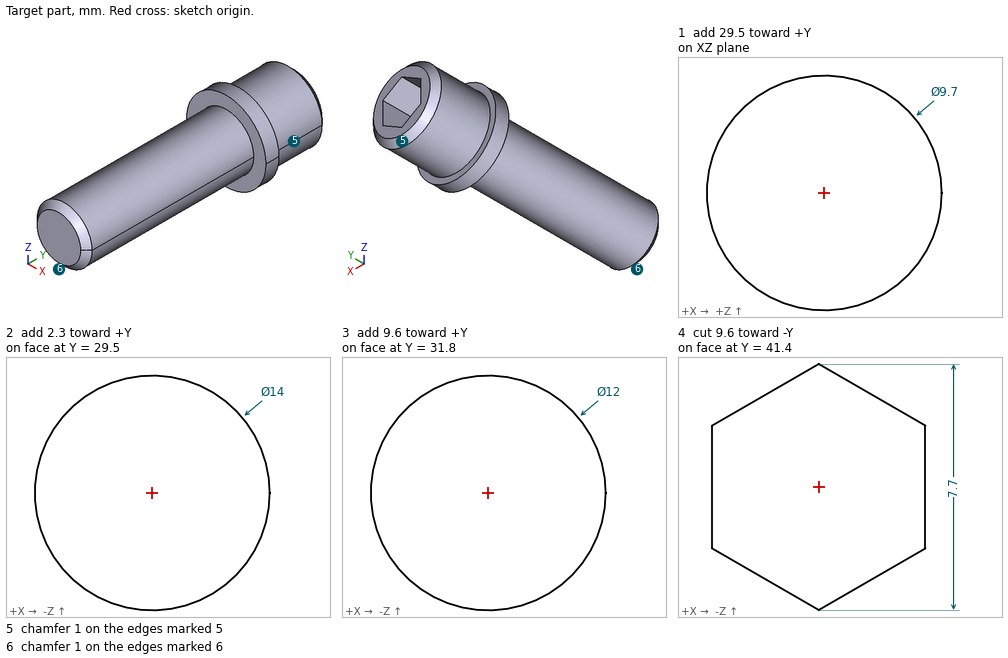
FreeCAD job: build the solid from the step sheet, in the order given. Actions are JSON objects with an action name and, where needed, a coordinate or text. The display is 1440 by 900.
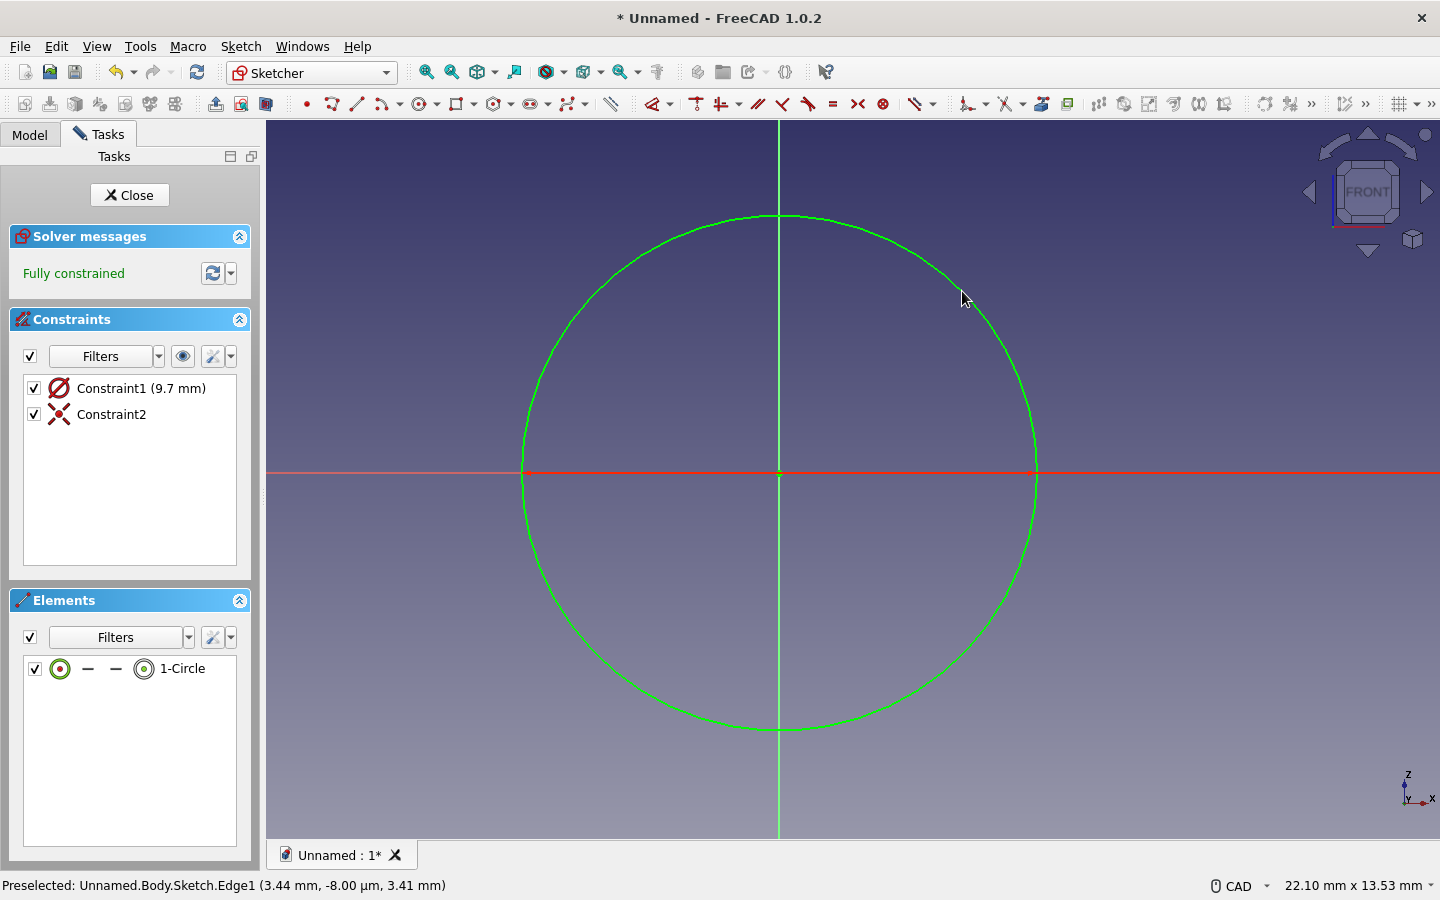
{"action": "left_click", "coordinate": [130, 195]}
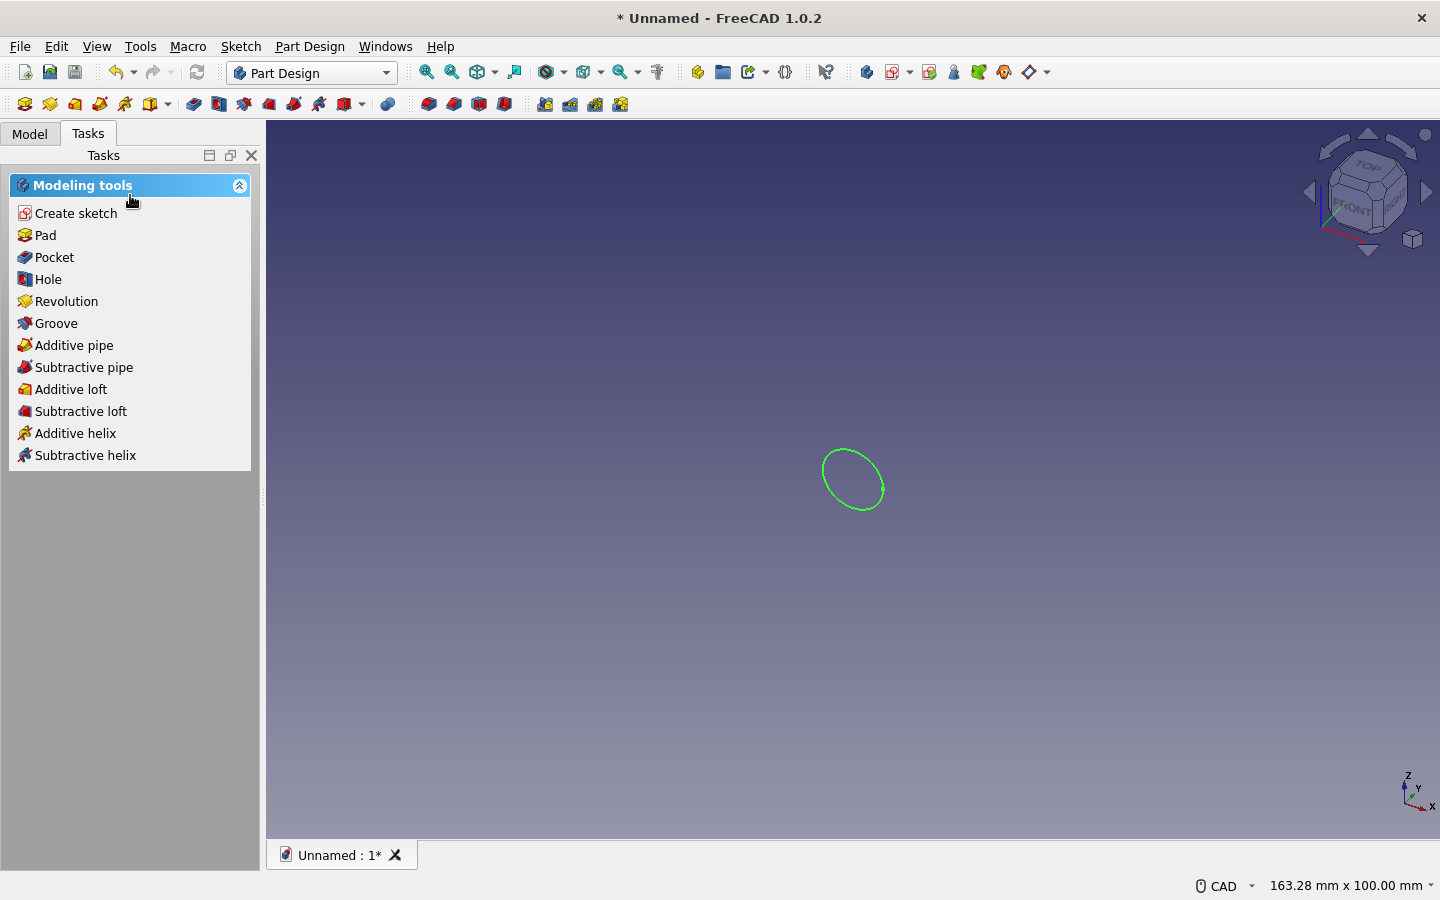
{"action": "left_click", "coordinate": [25, 104]}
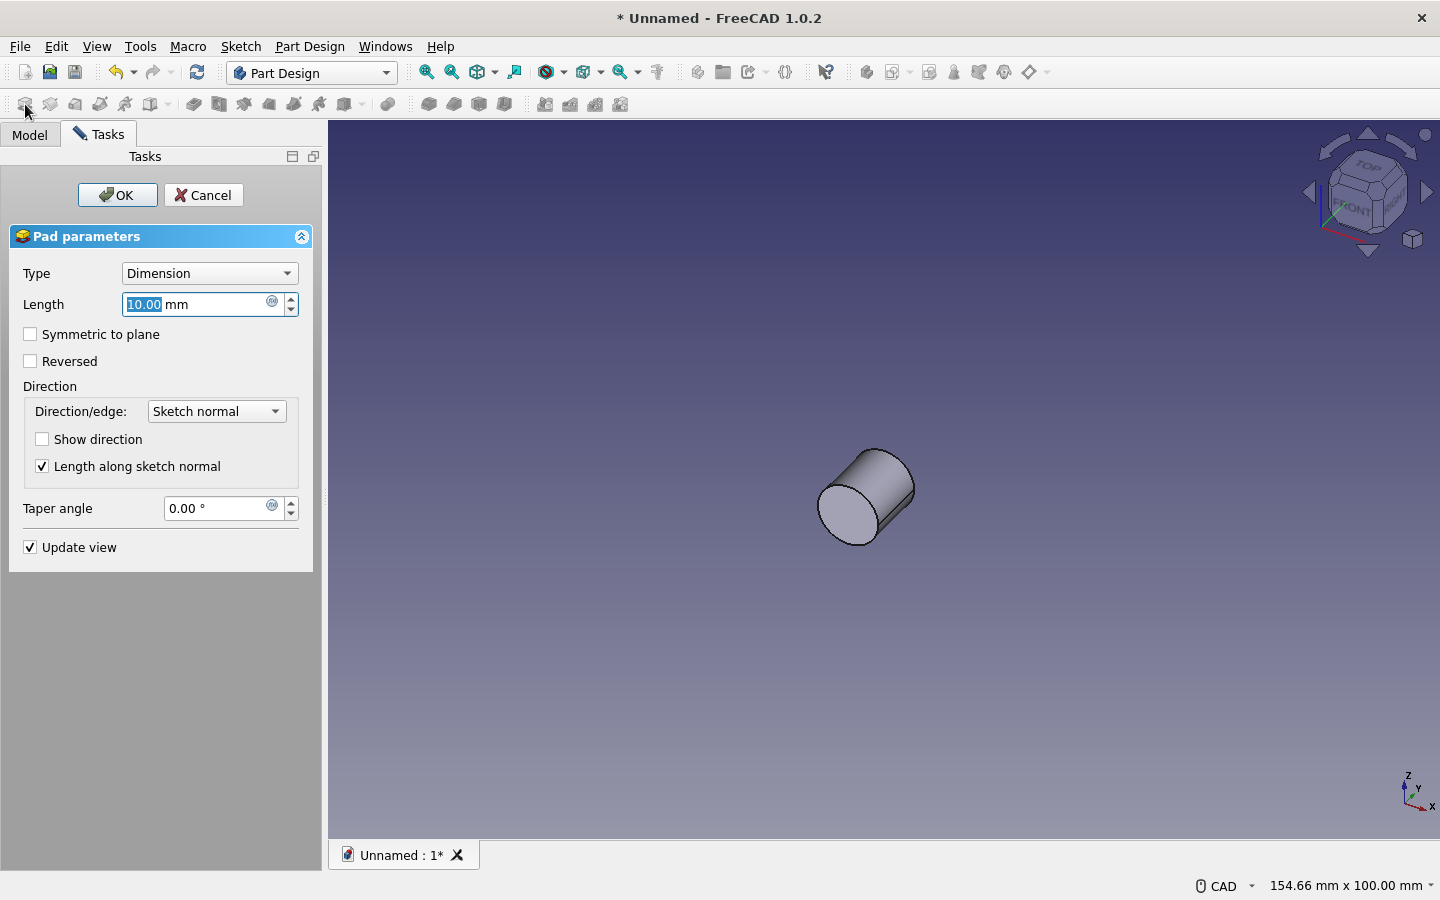
{"action": "type", "text": "29.5"}
{"action": "key", "text": "Tab"}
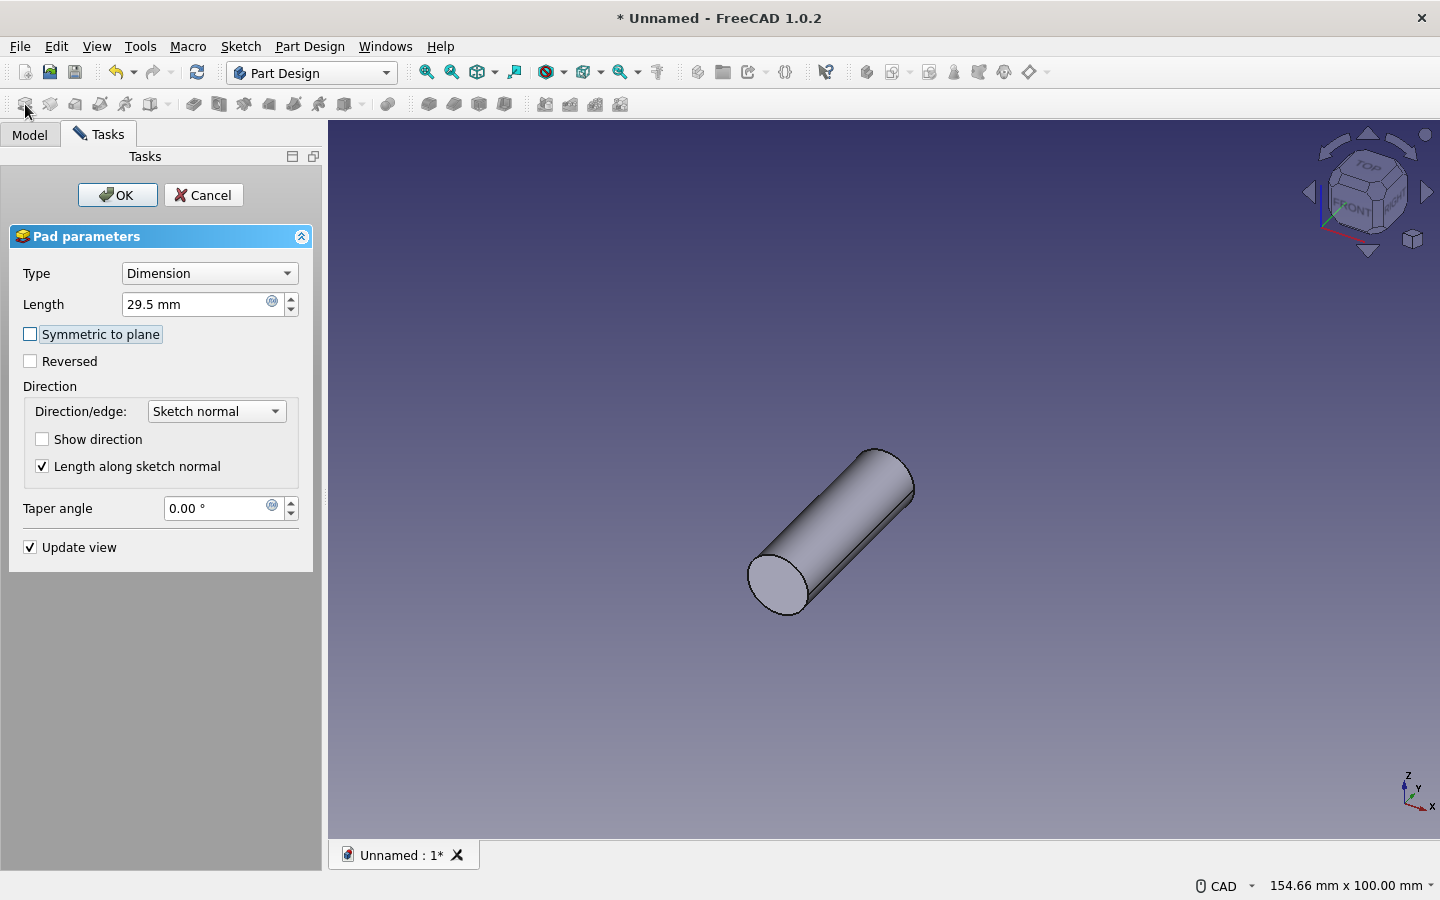
{"action": "left_click", "coordinate": [31, 361]}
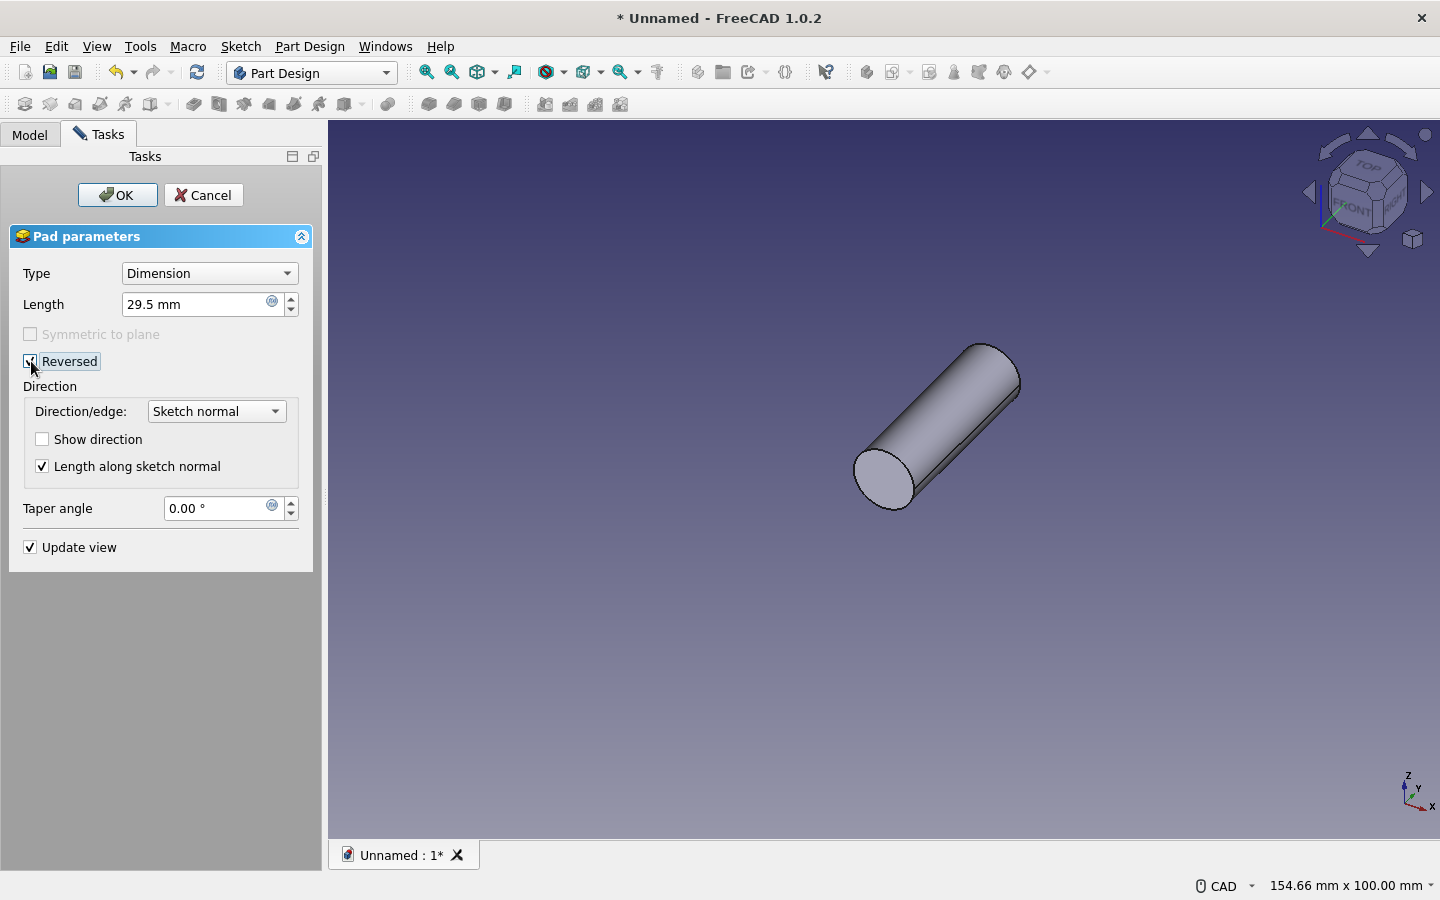
{"action": "left_click", "coordinate": [118, 195]}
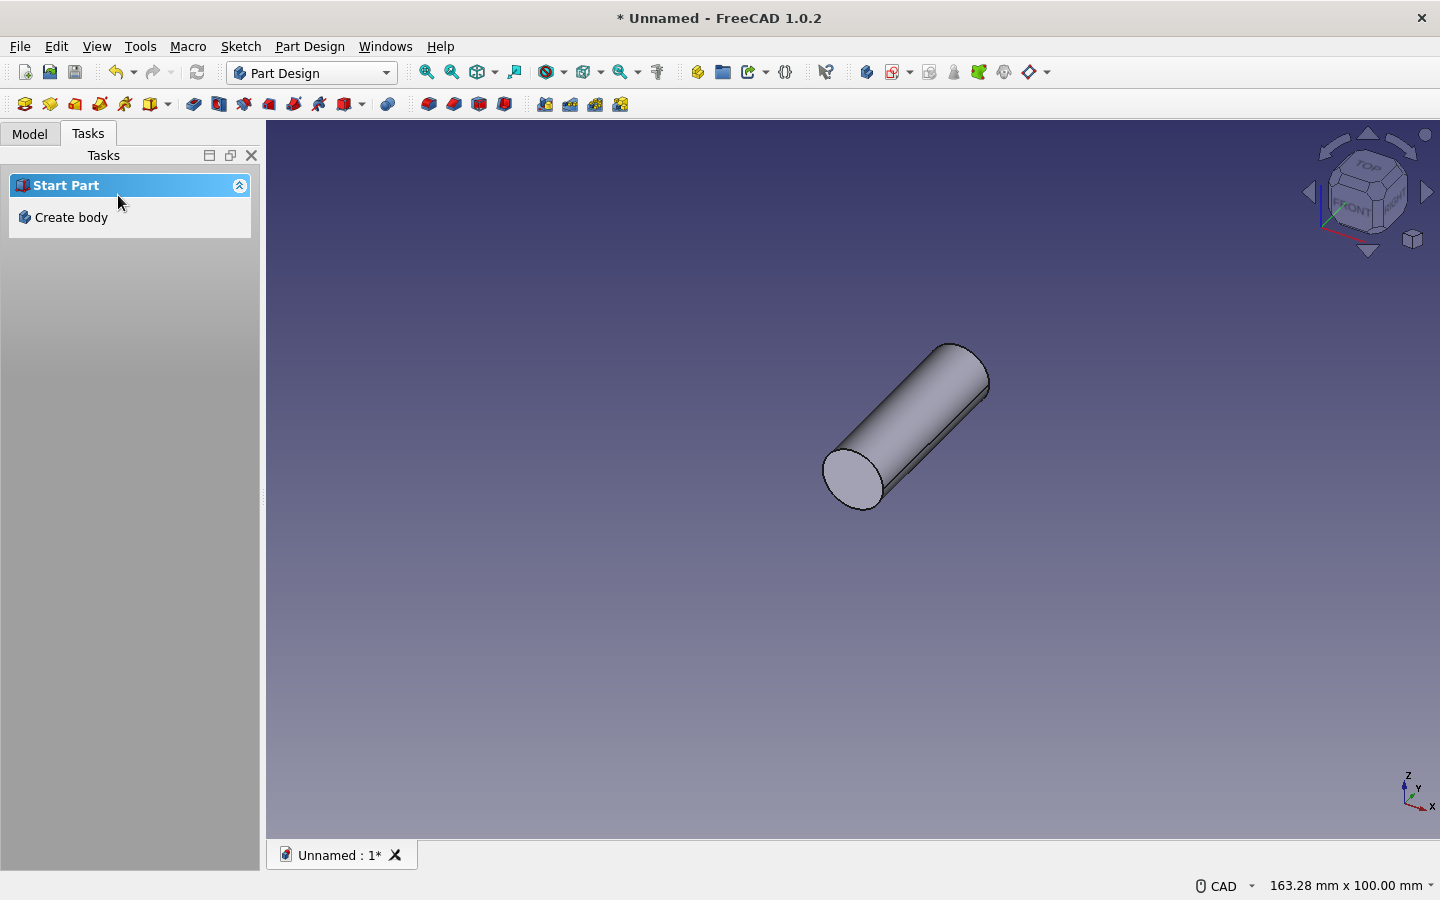
{"action": "left_click", "coordinate": [427, 72]}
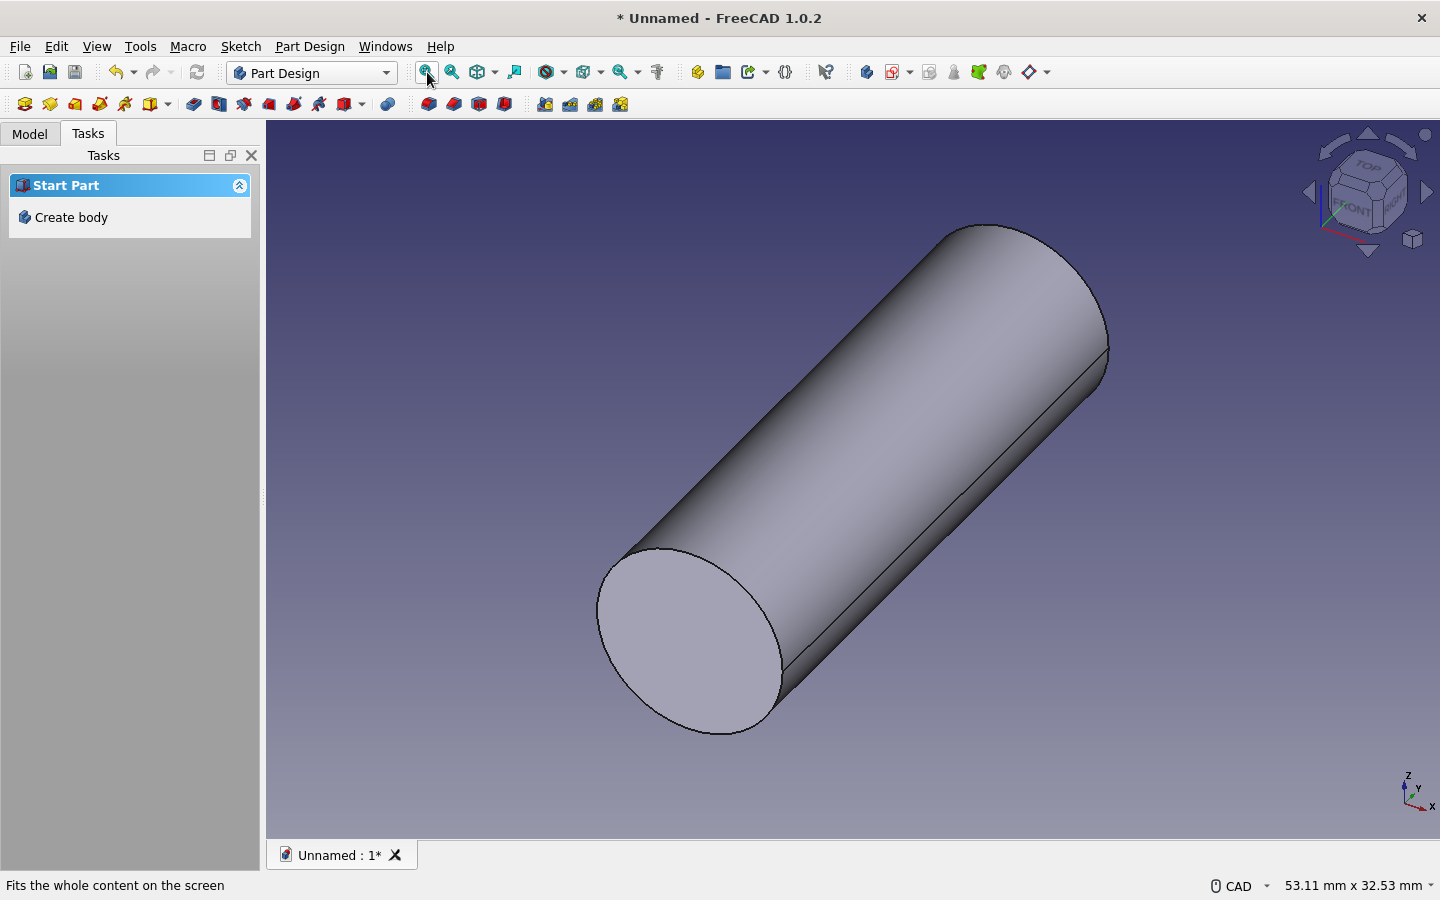
{"action": "key", "text": "4"}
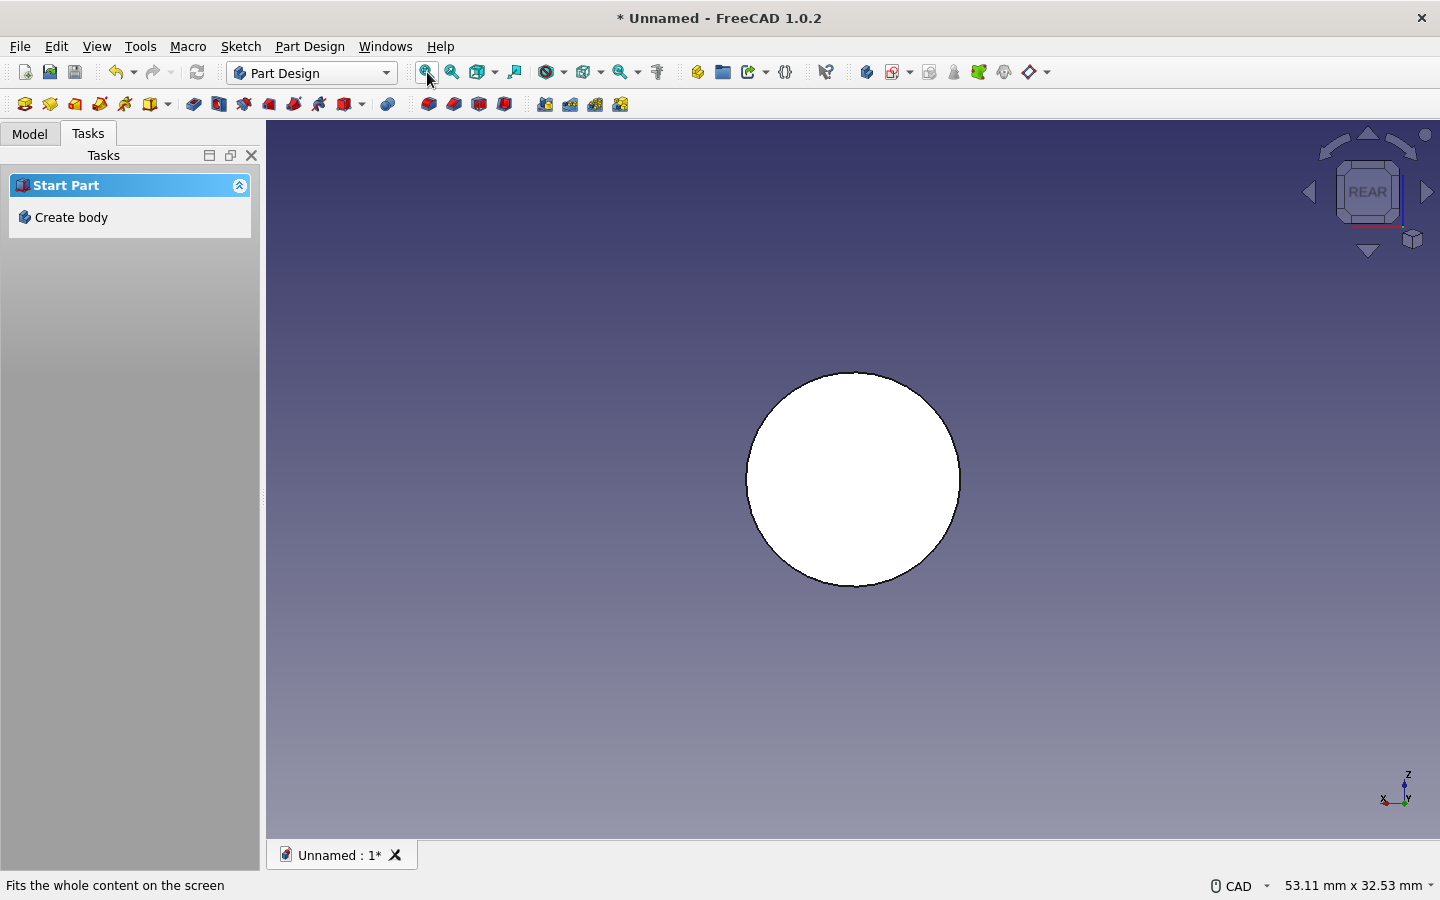
{"action": "left_click", "coordinate": [427, 72]}